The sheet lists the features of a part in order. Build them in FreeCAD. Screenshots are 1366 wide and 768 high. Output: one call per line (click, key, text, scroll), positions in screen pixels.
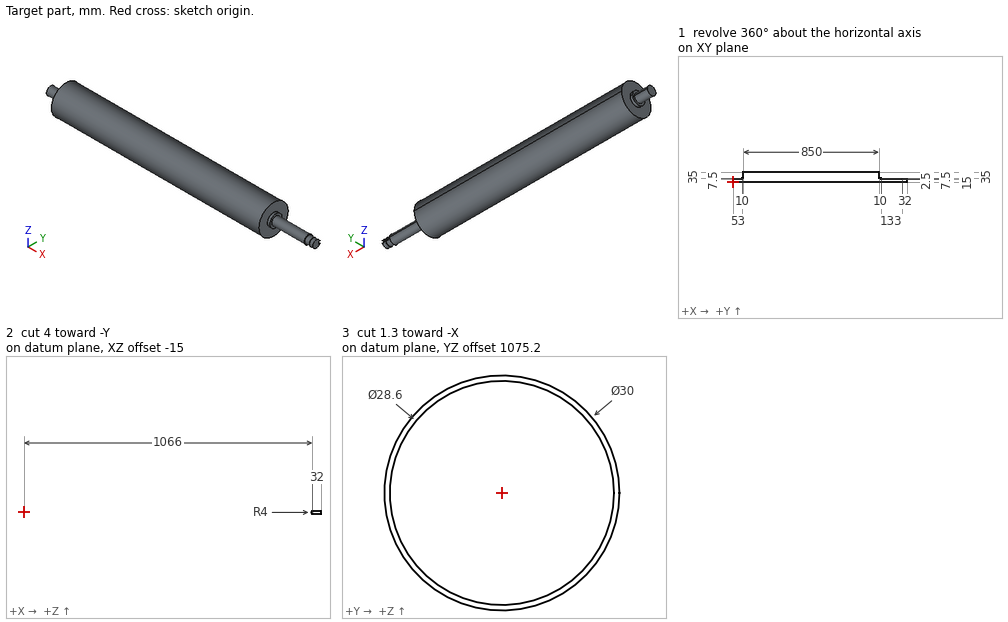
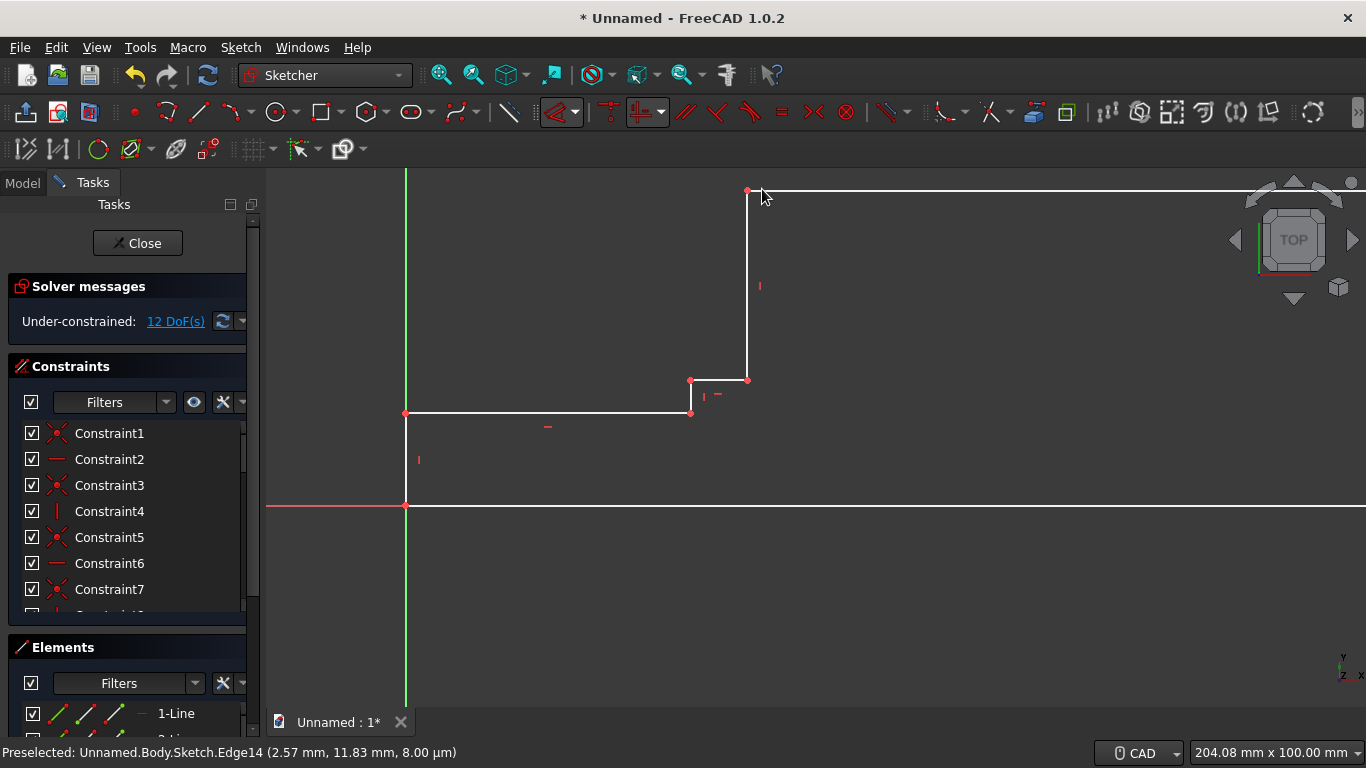
scroll(425, 449, down, 11)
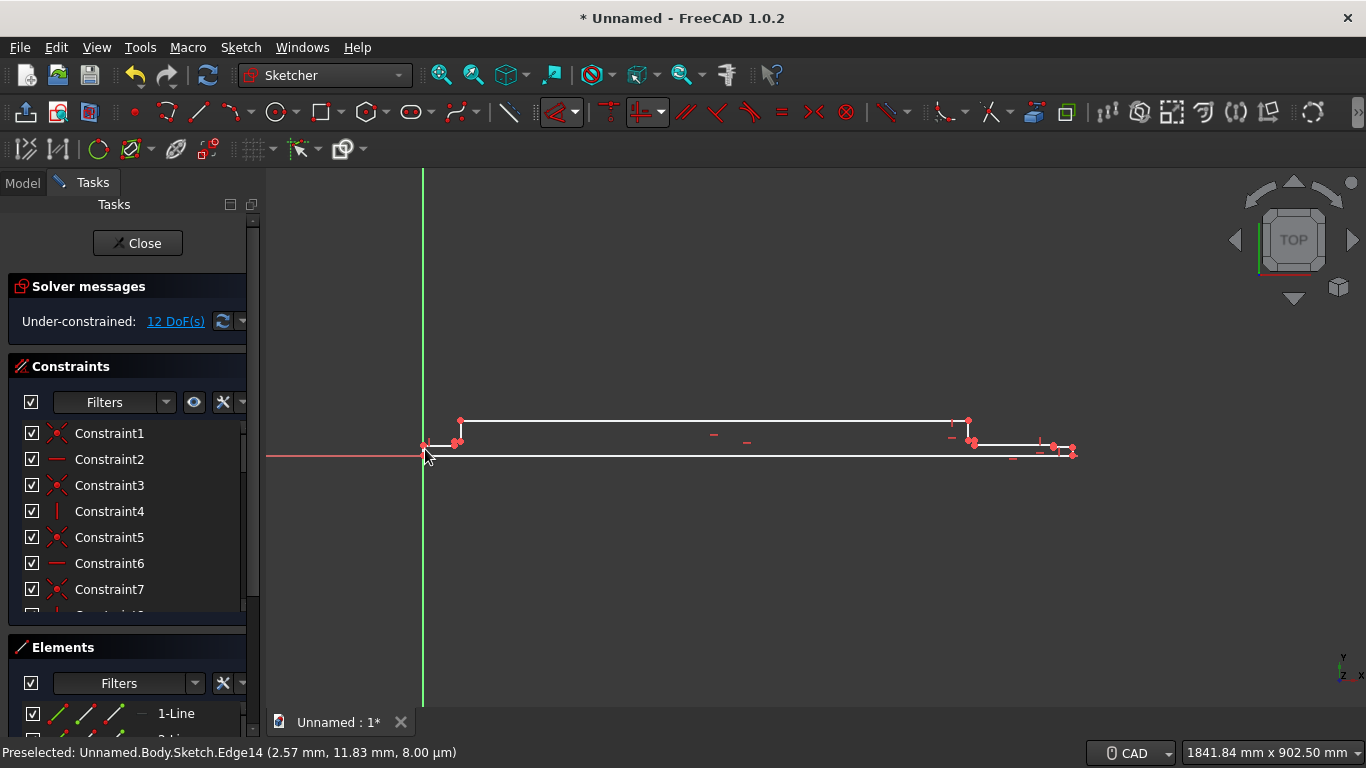
scroll(1073, 453, up, 9)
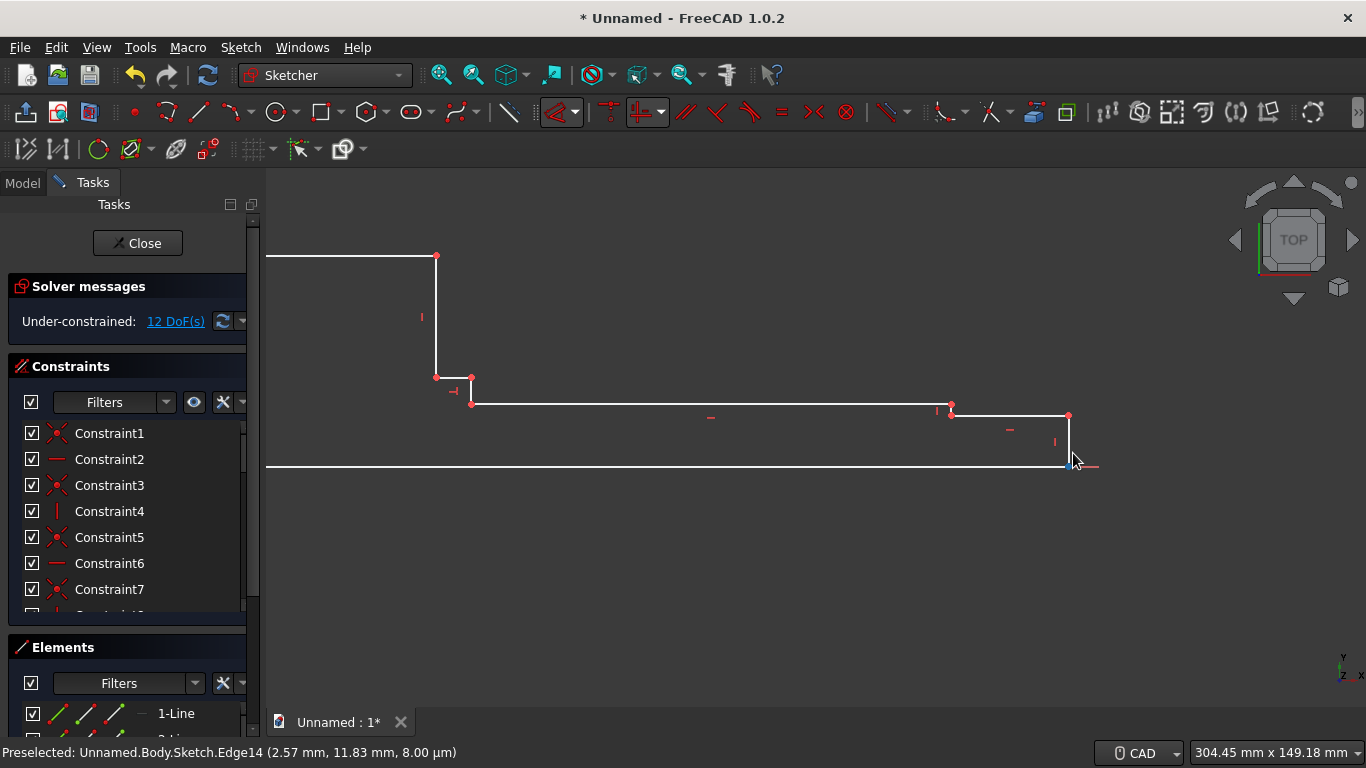
click(1069, 452)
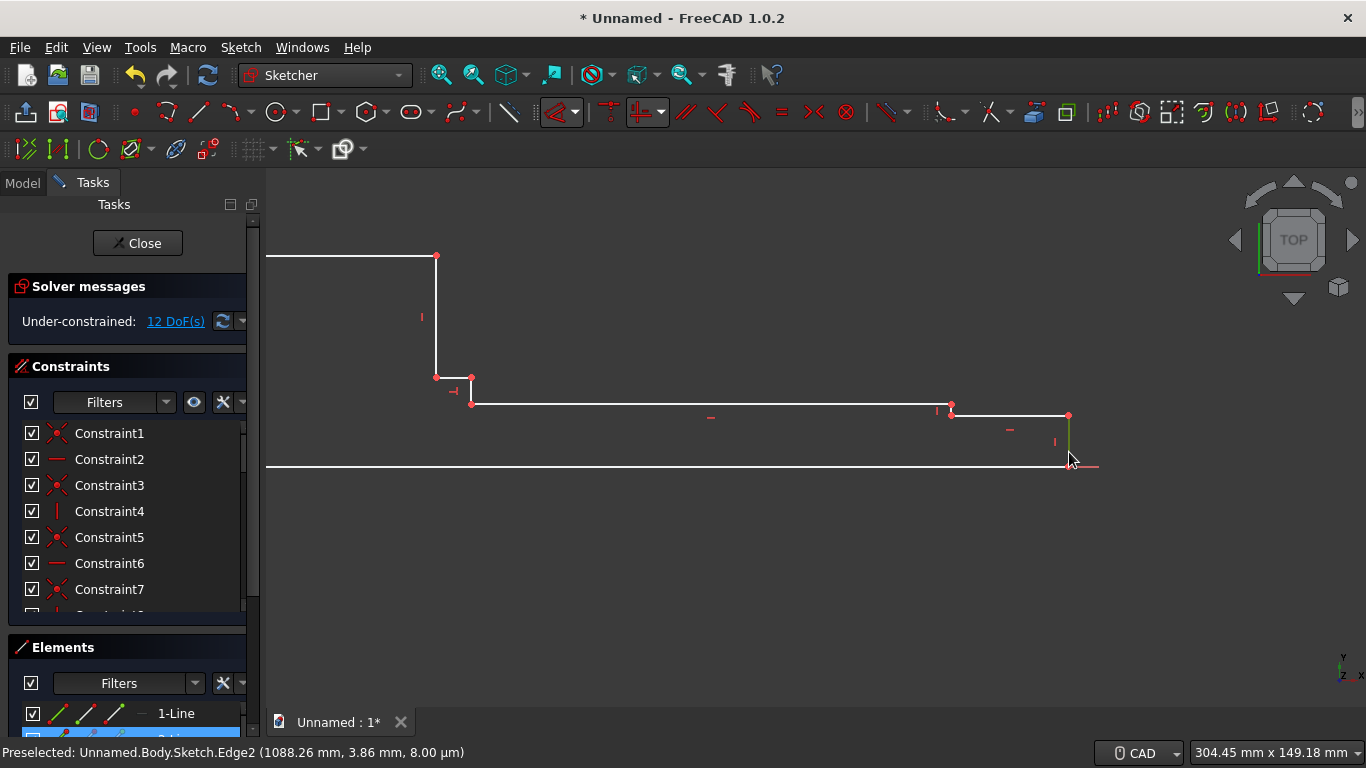
key(i)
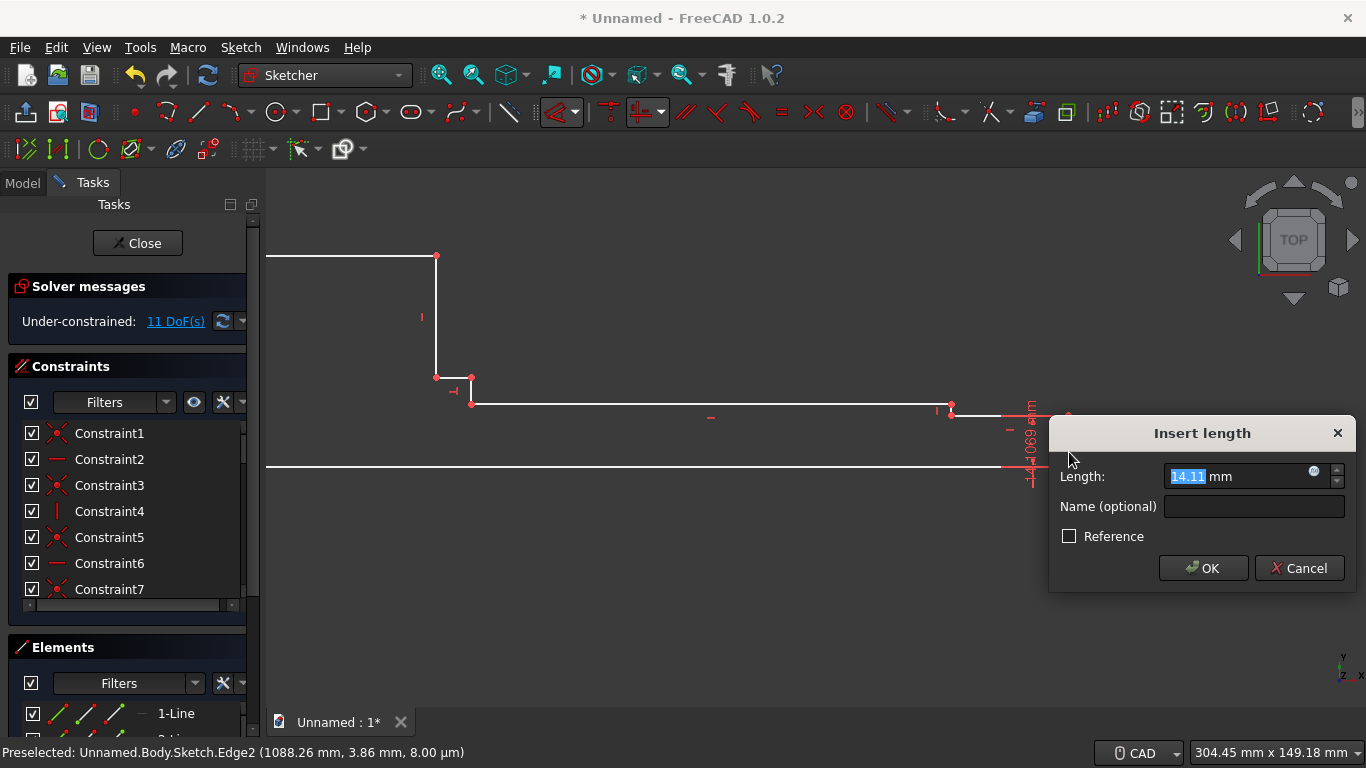
text(15)
key(Return)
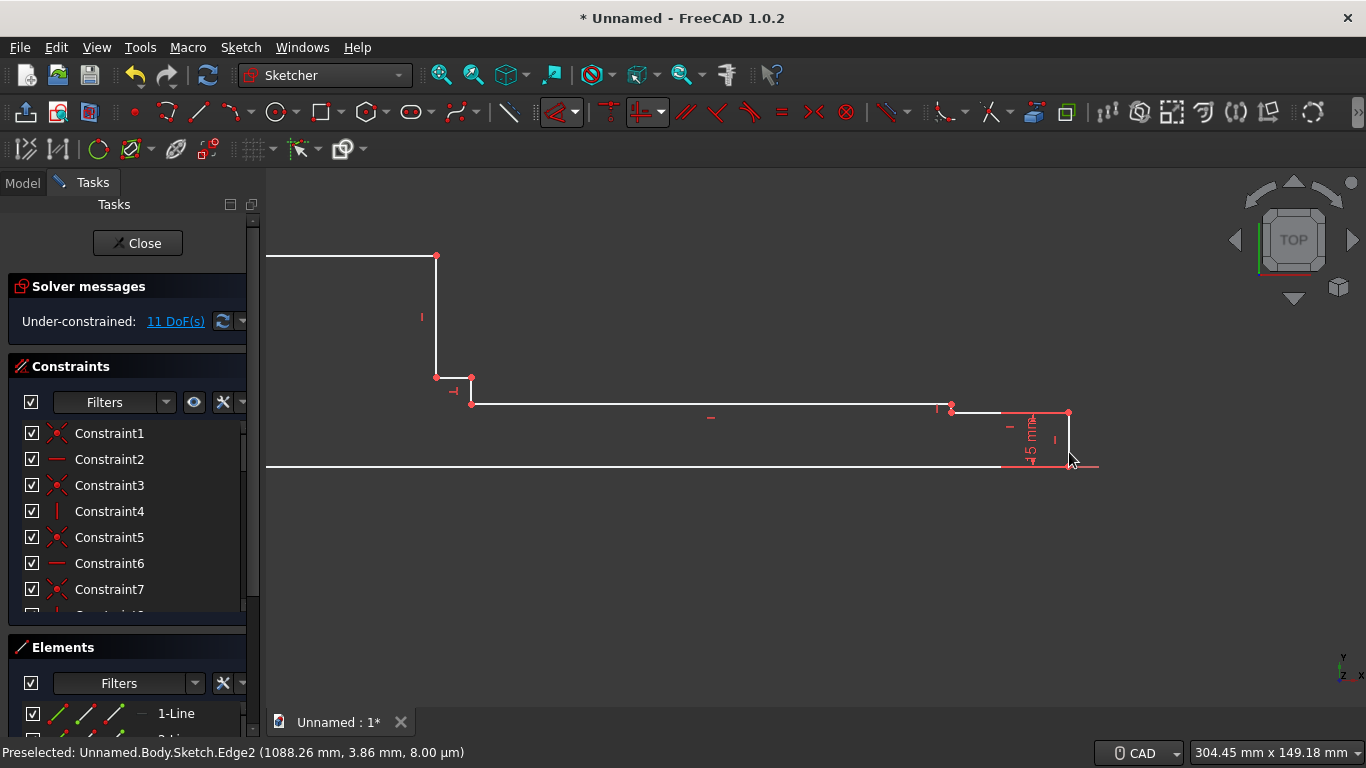
click(1034, 413)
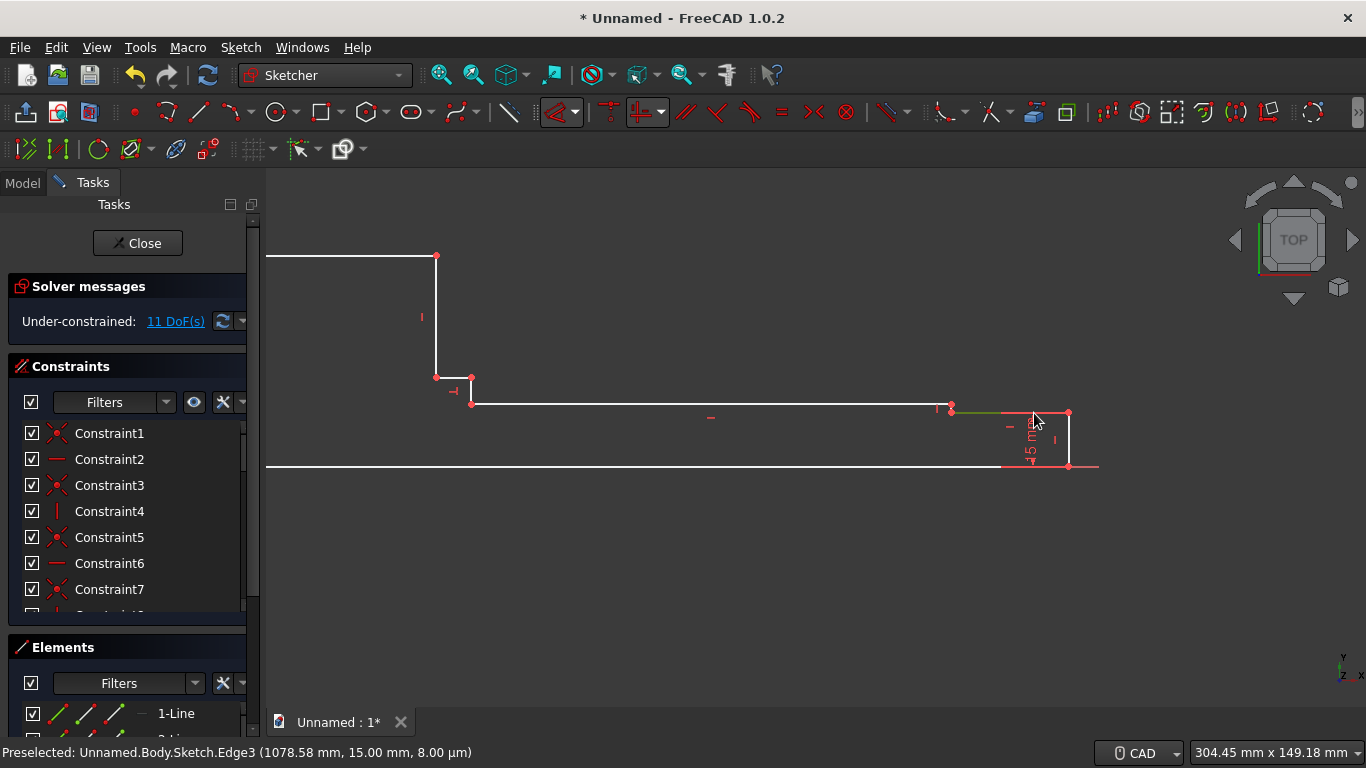
click(578, 112)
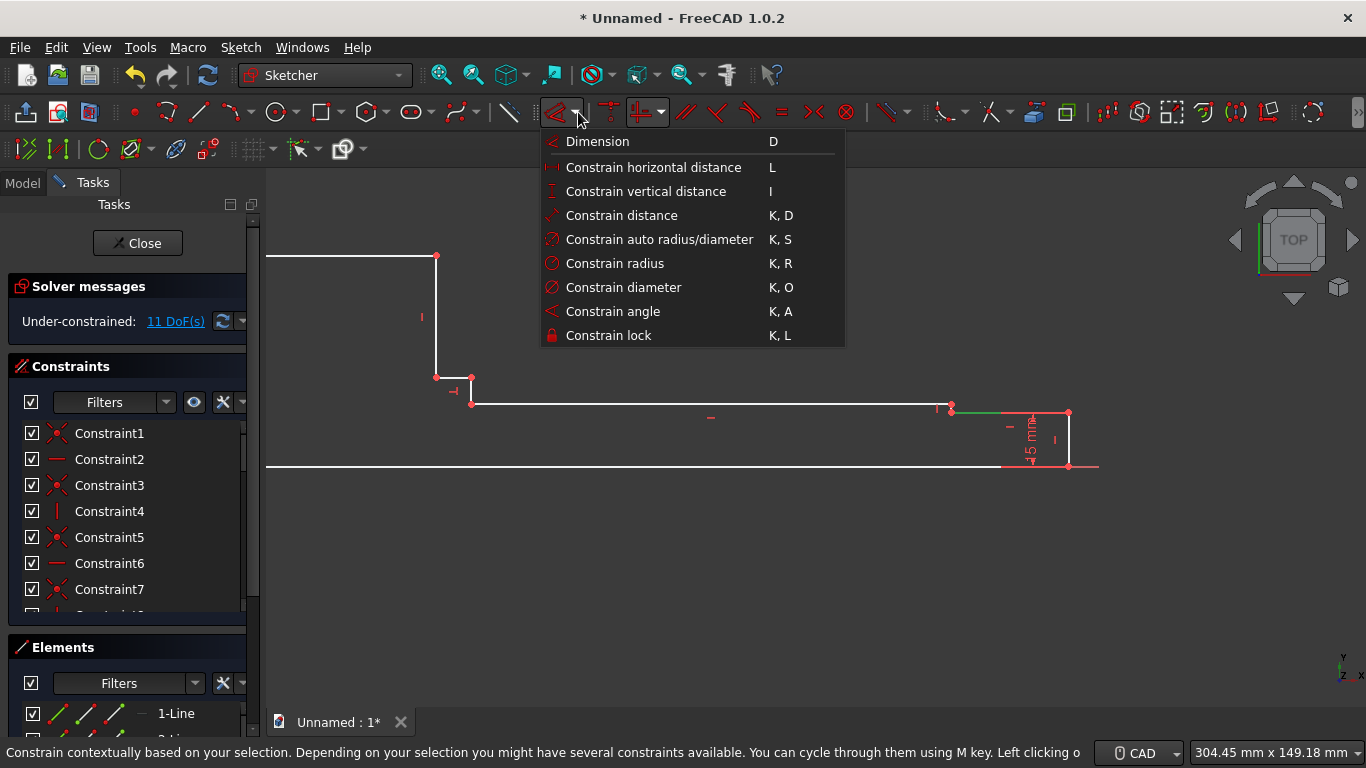
click(693, 167)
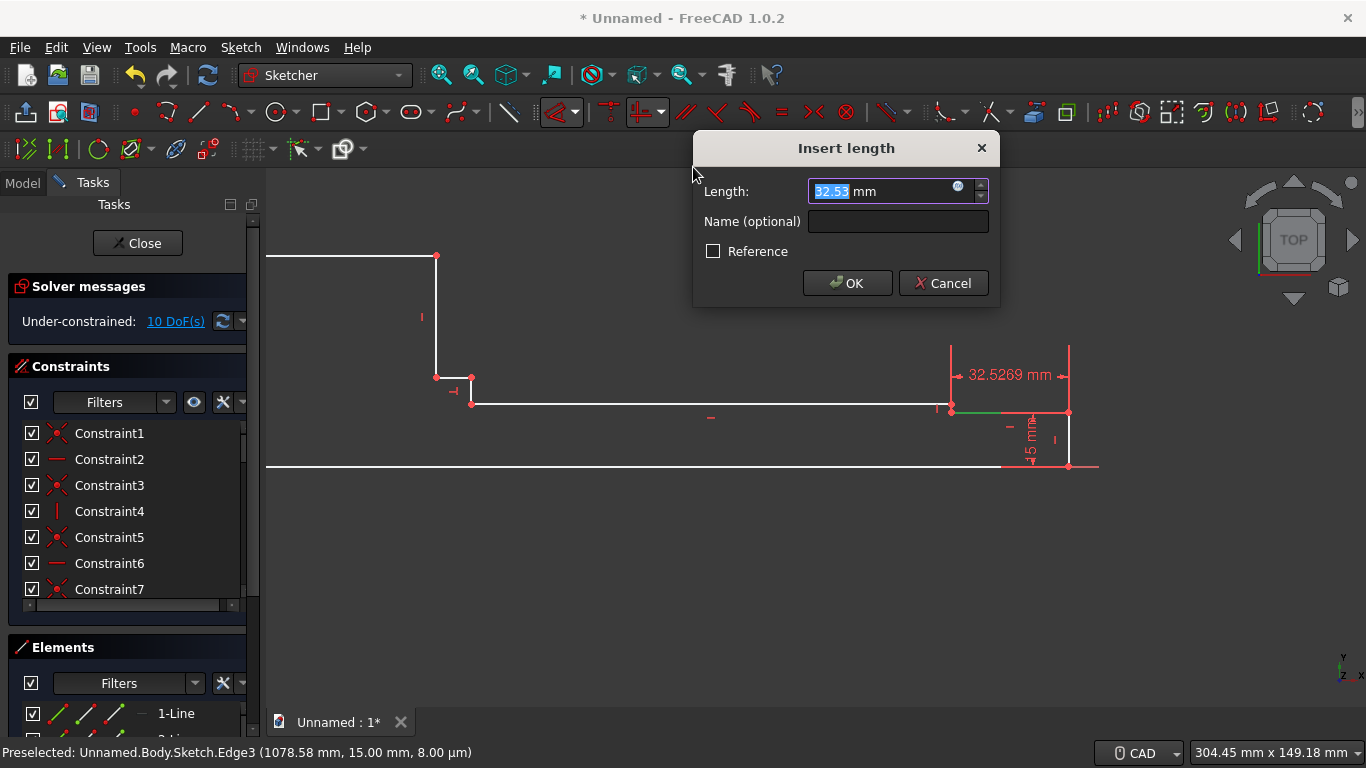
text(32)
key(Return)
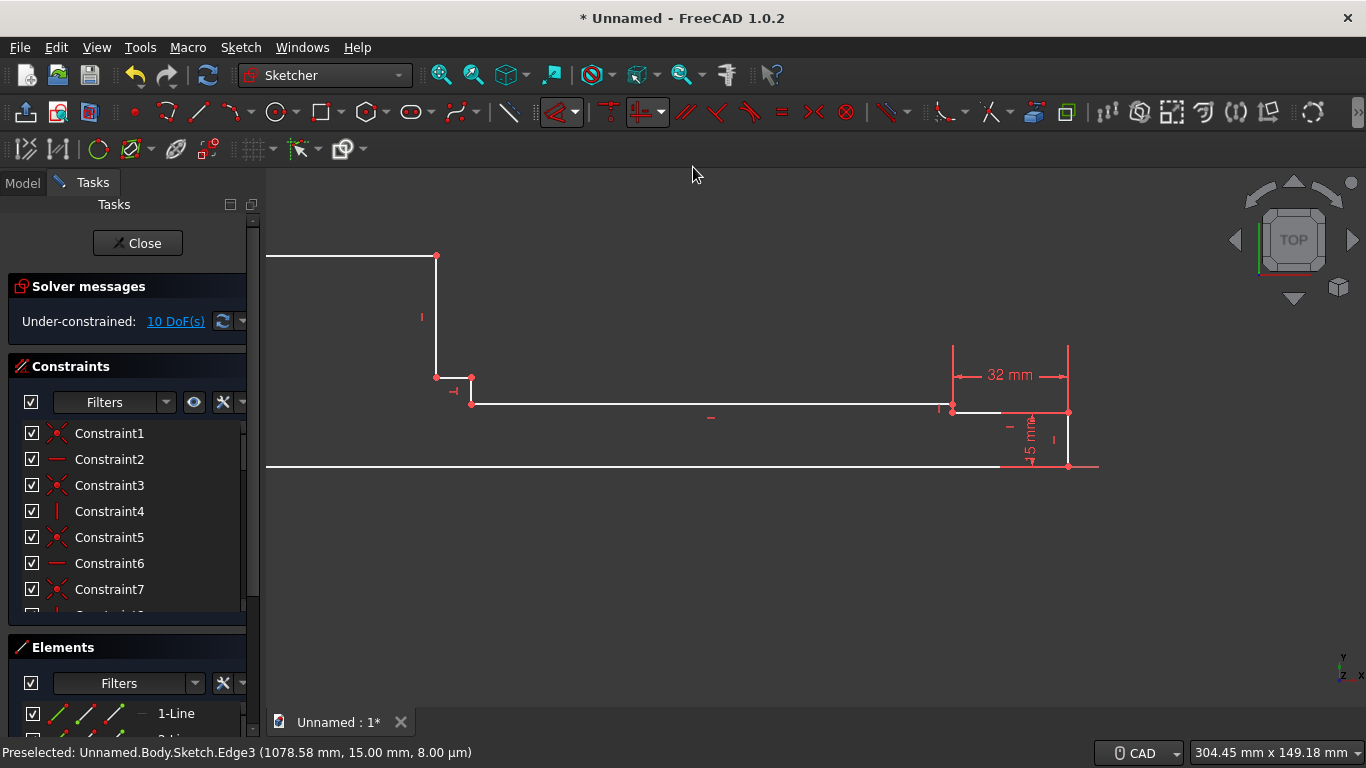
scroll(461, 378, up, 2)